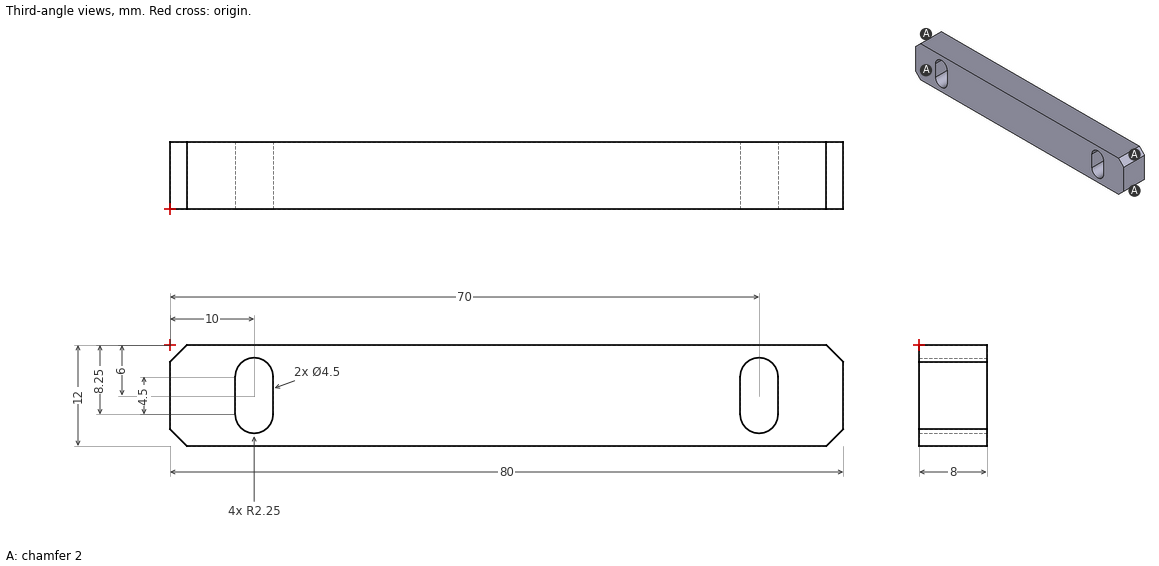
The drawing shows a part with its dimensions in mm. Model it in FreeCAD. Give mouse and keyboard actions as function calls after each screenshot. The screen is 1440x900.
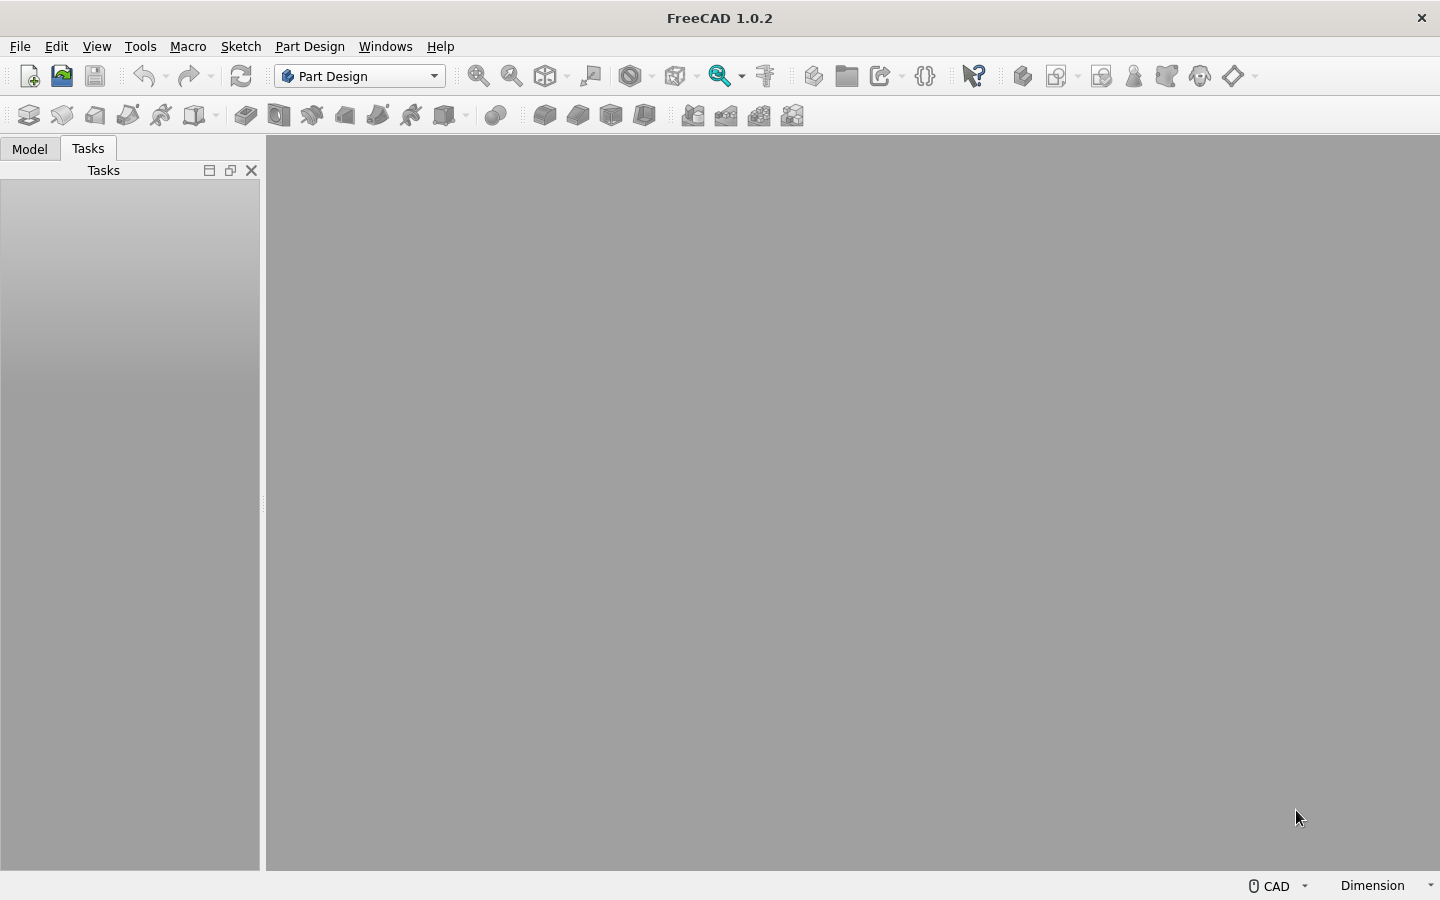
key(ctrl+n)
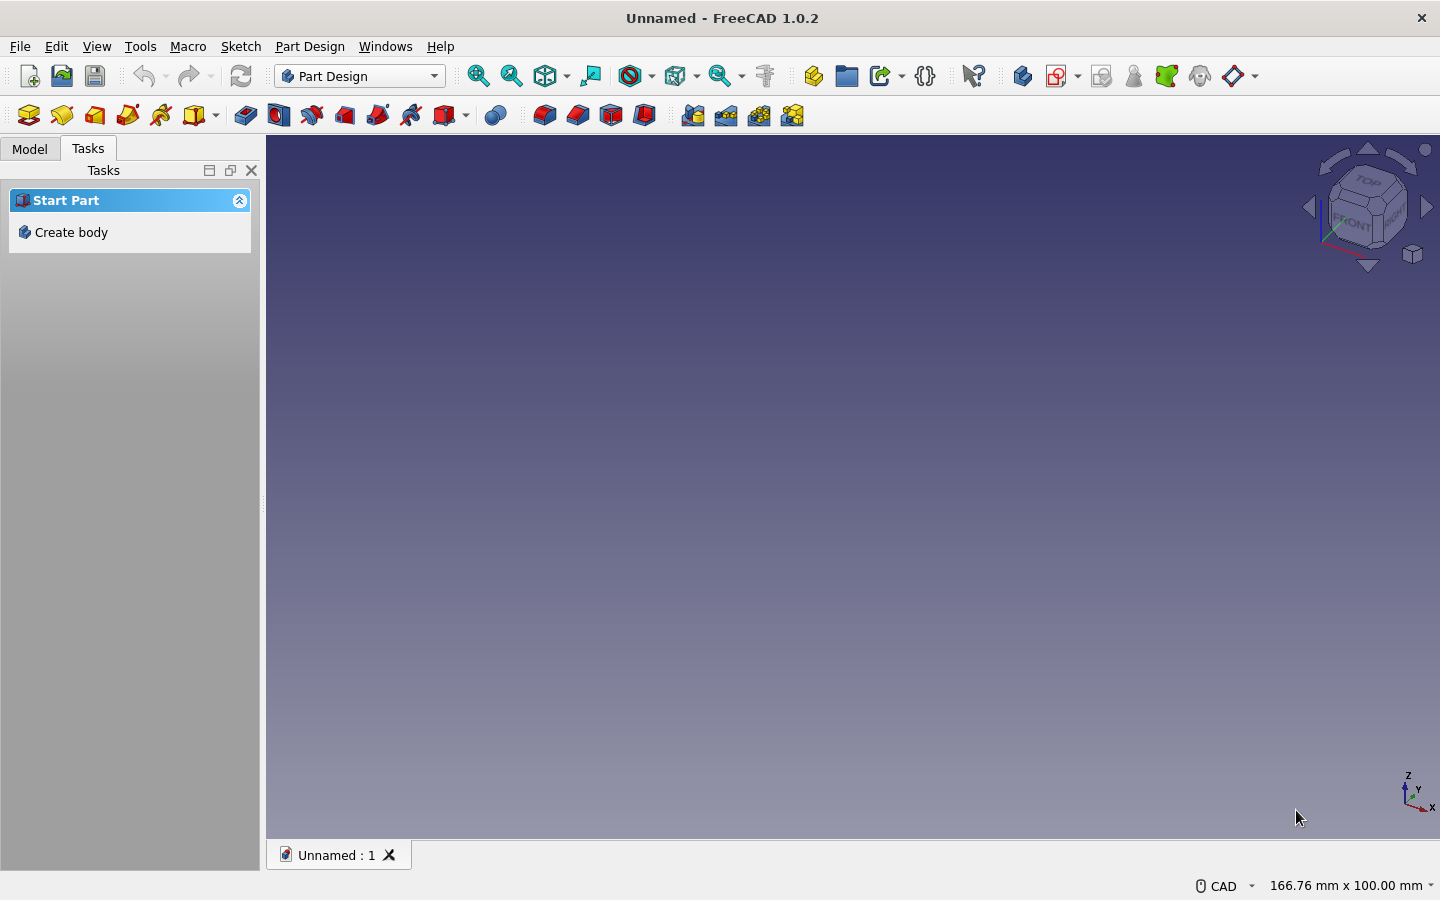
click(1056, 76)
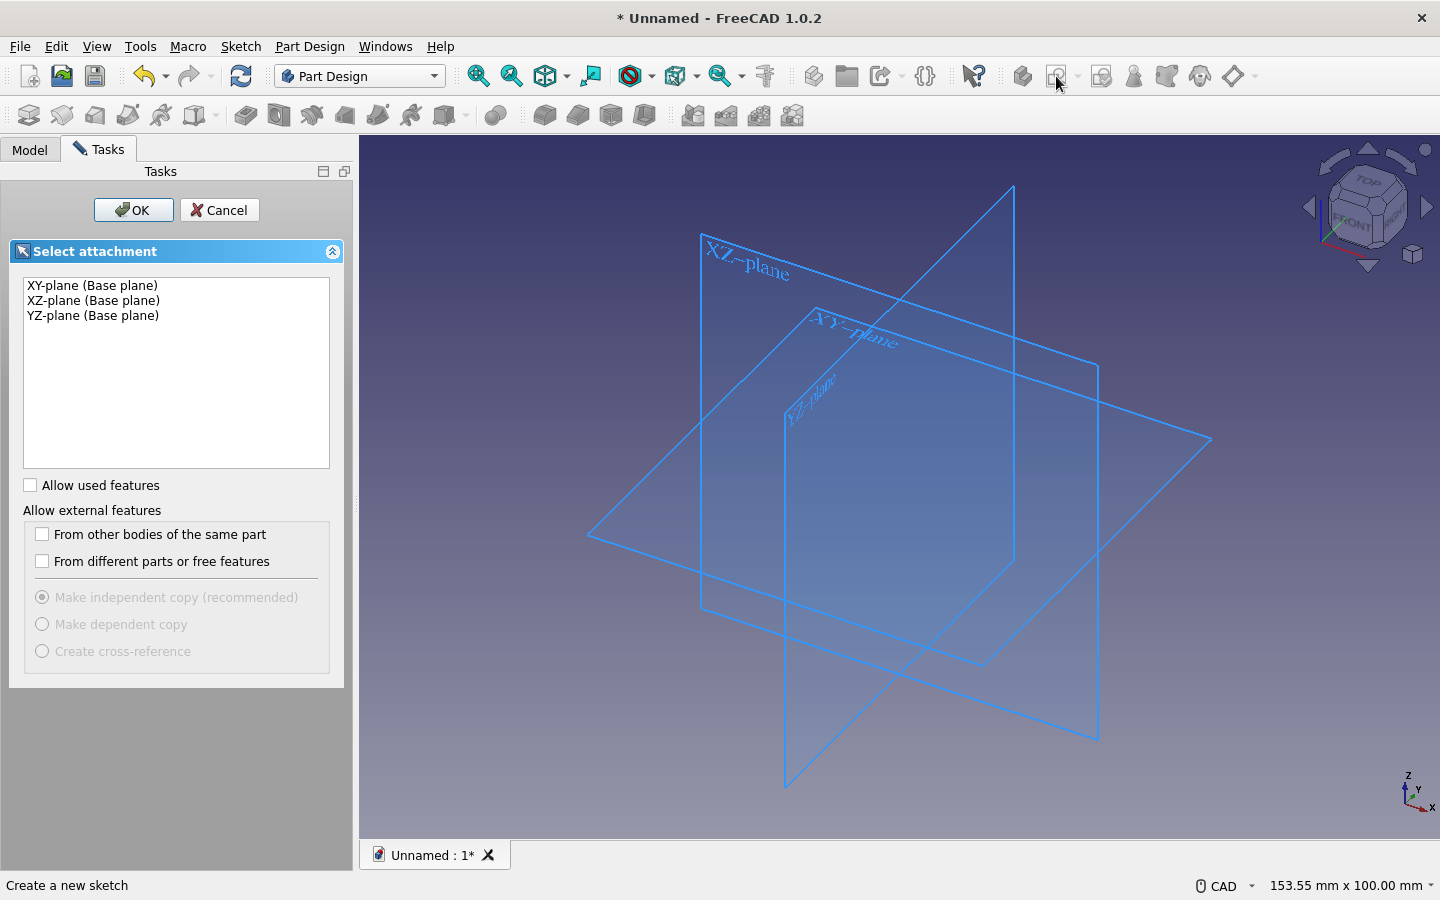
click(84, 300)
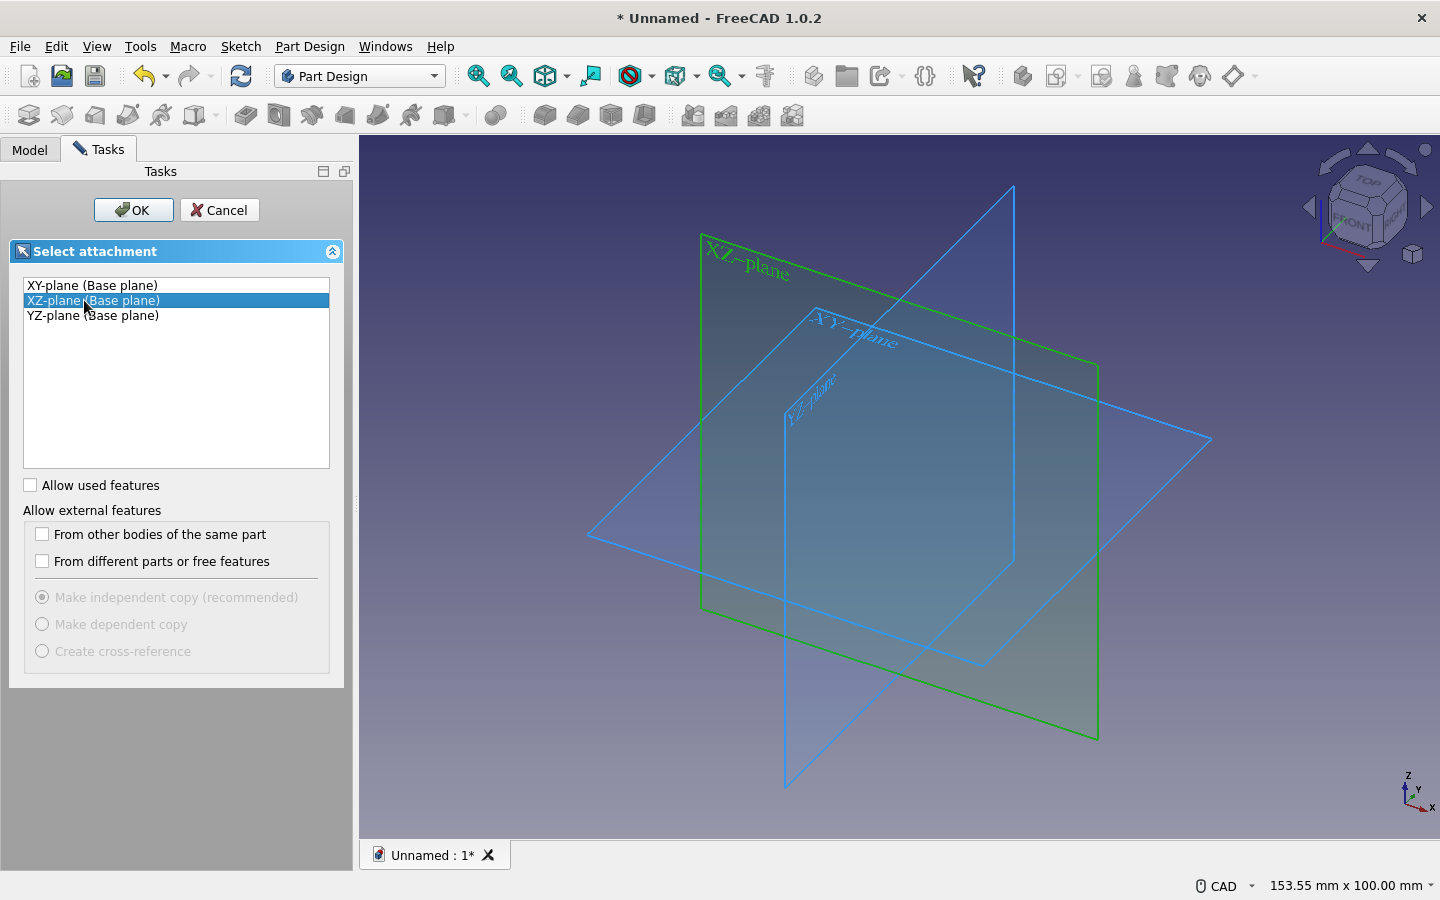
click(134, 210)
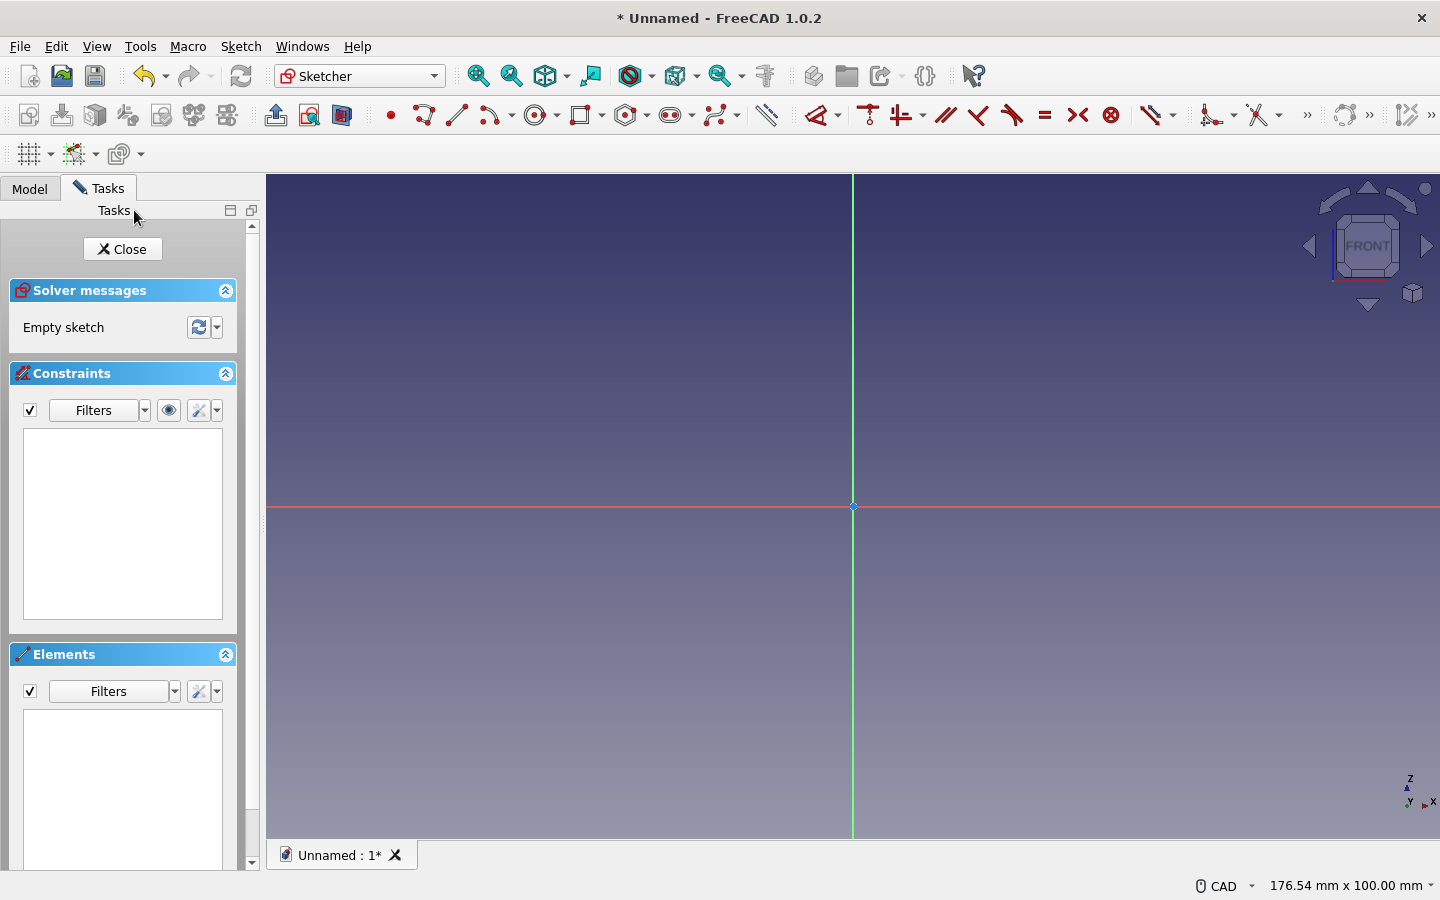
scroll(294, 326, down, 1)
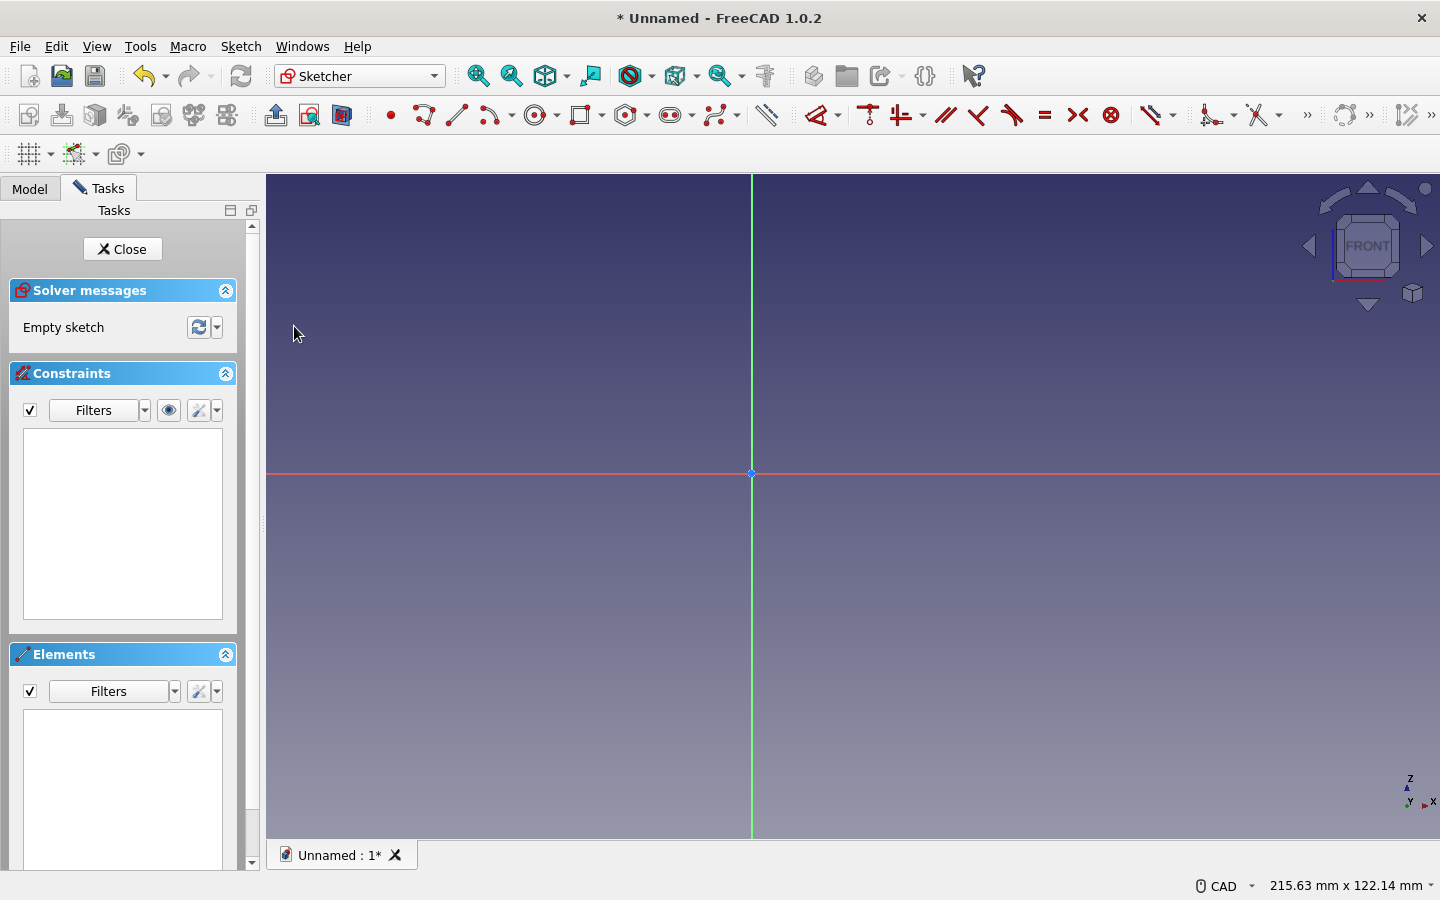
scroll(1275, 506, up, 2)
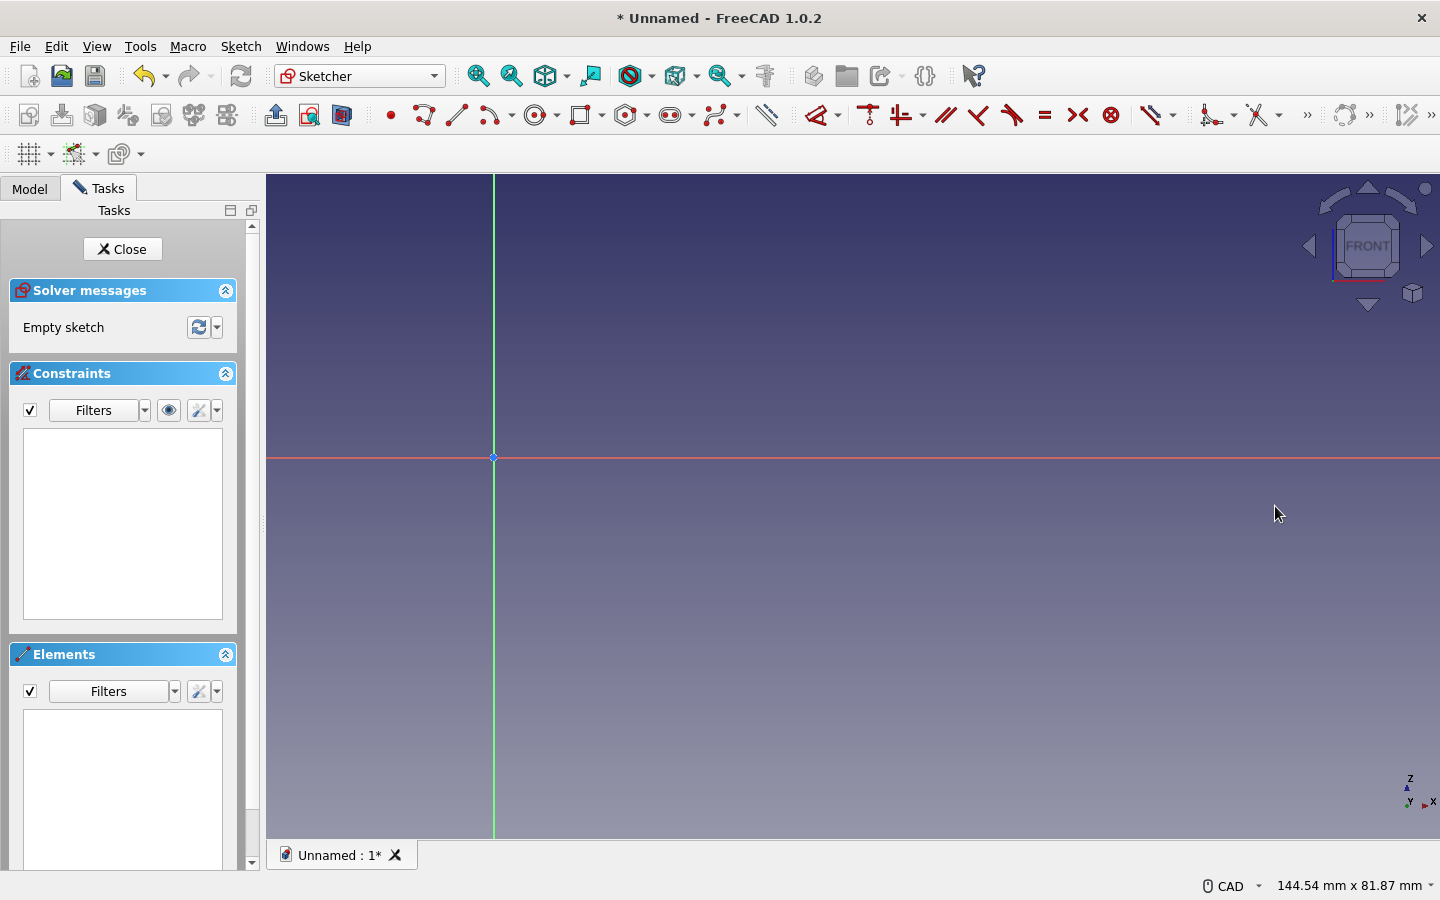
key(g)
key(r)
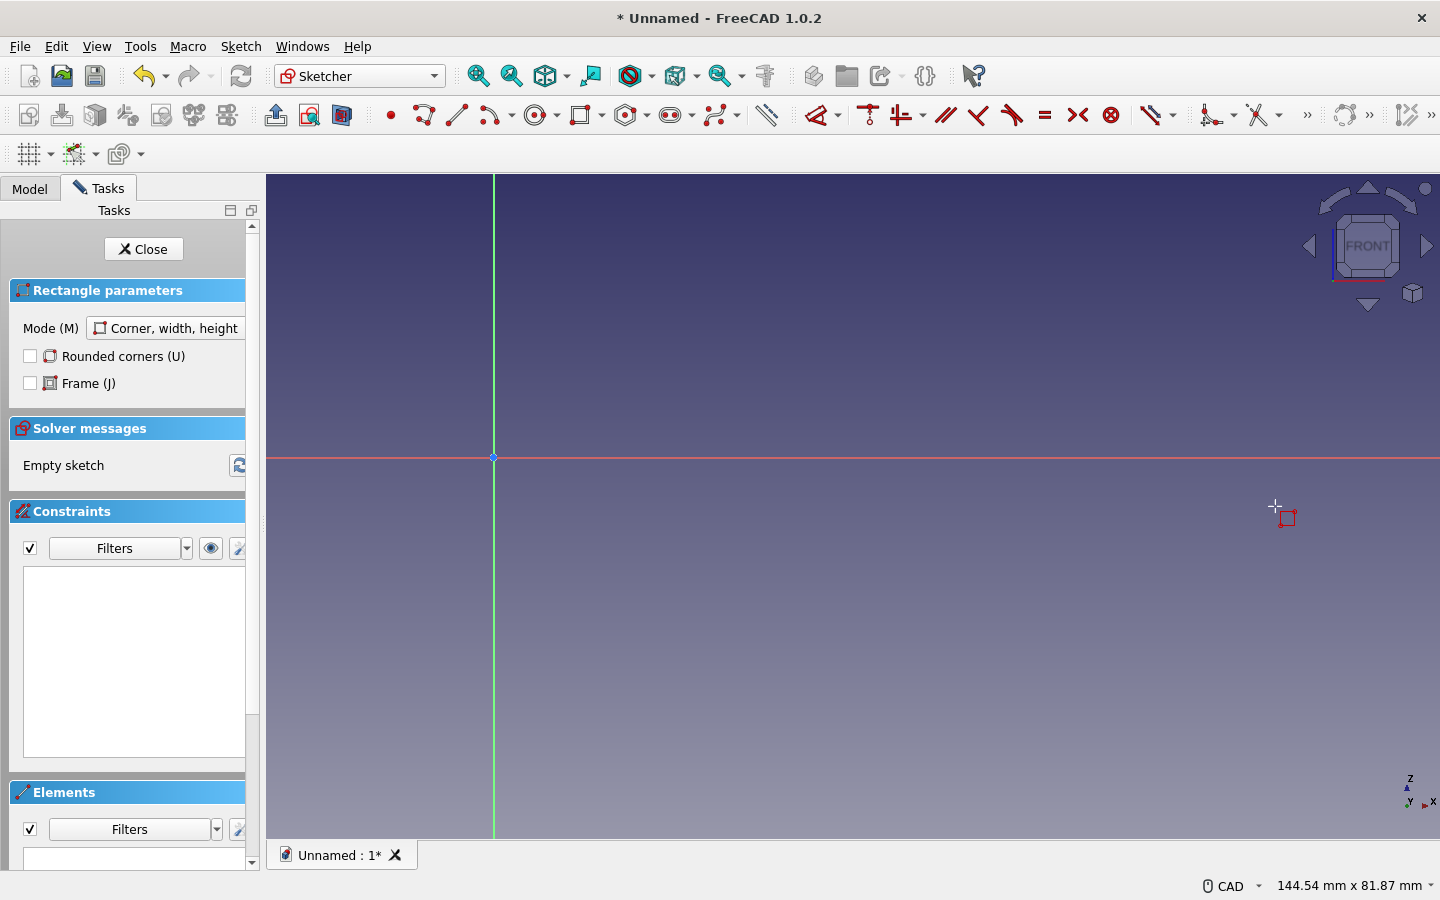
click(494, 458)
click(1144, 555)
key(Escape)